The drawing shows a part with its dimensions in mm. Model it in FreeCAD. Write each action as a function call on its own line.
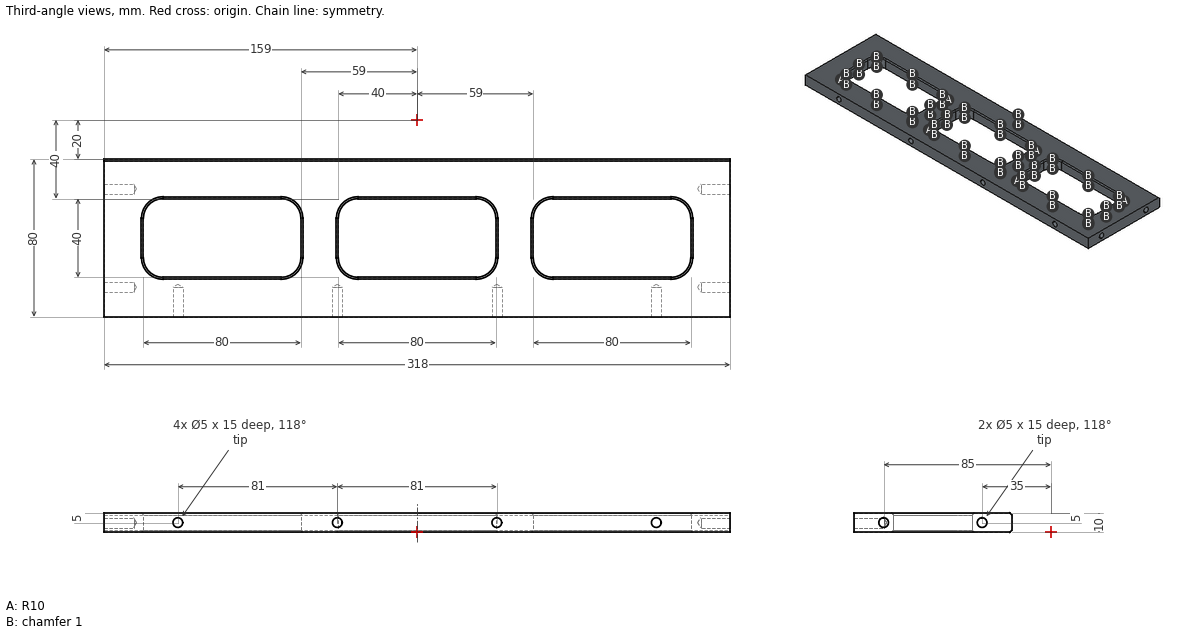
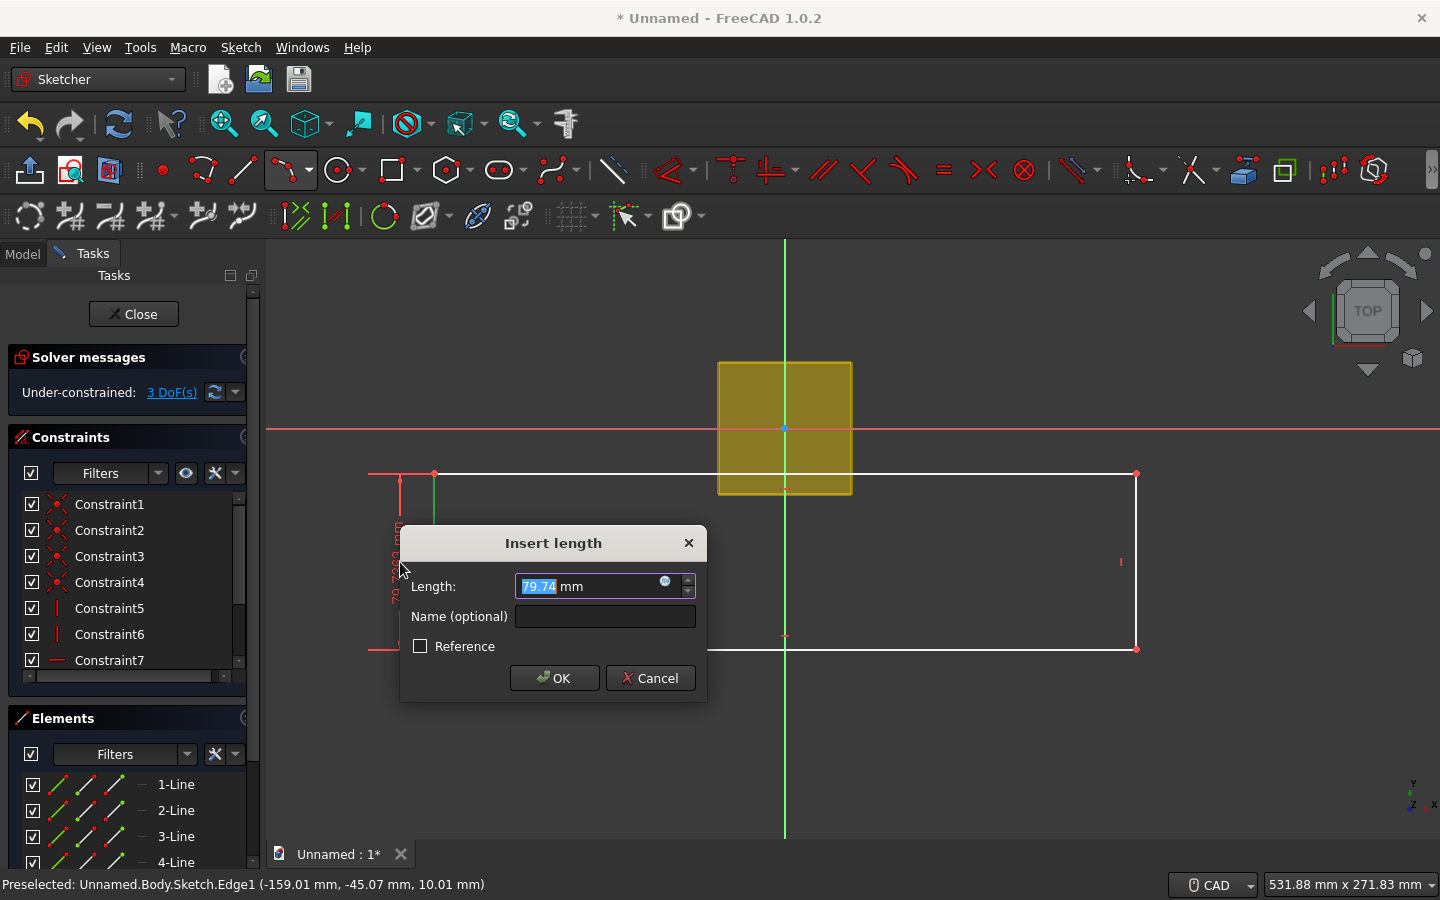
text(80)
key(Return)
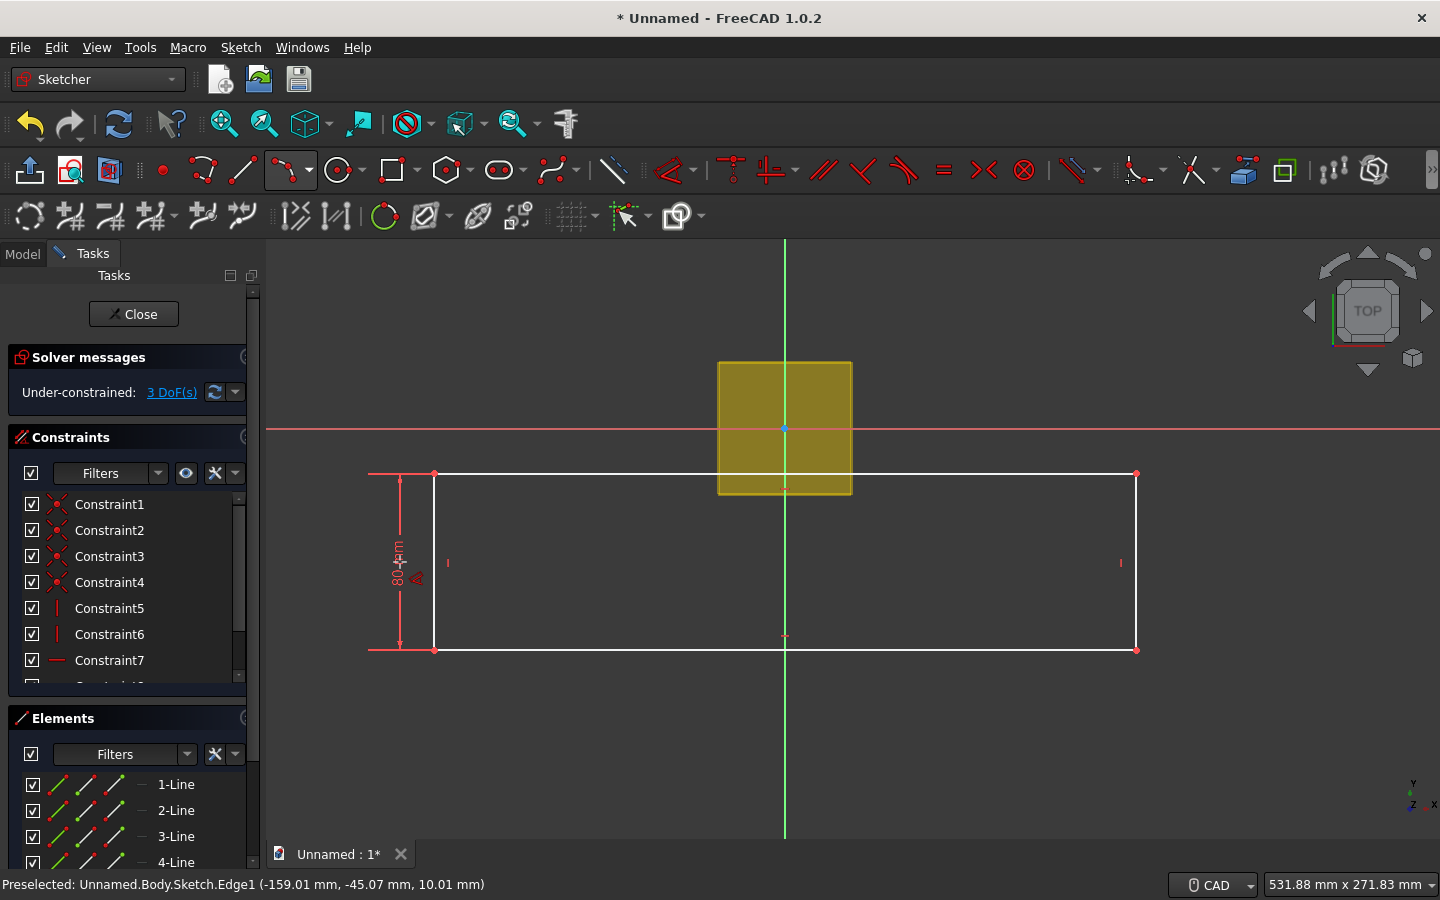
click(645, 650)
click(624, 684)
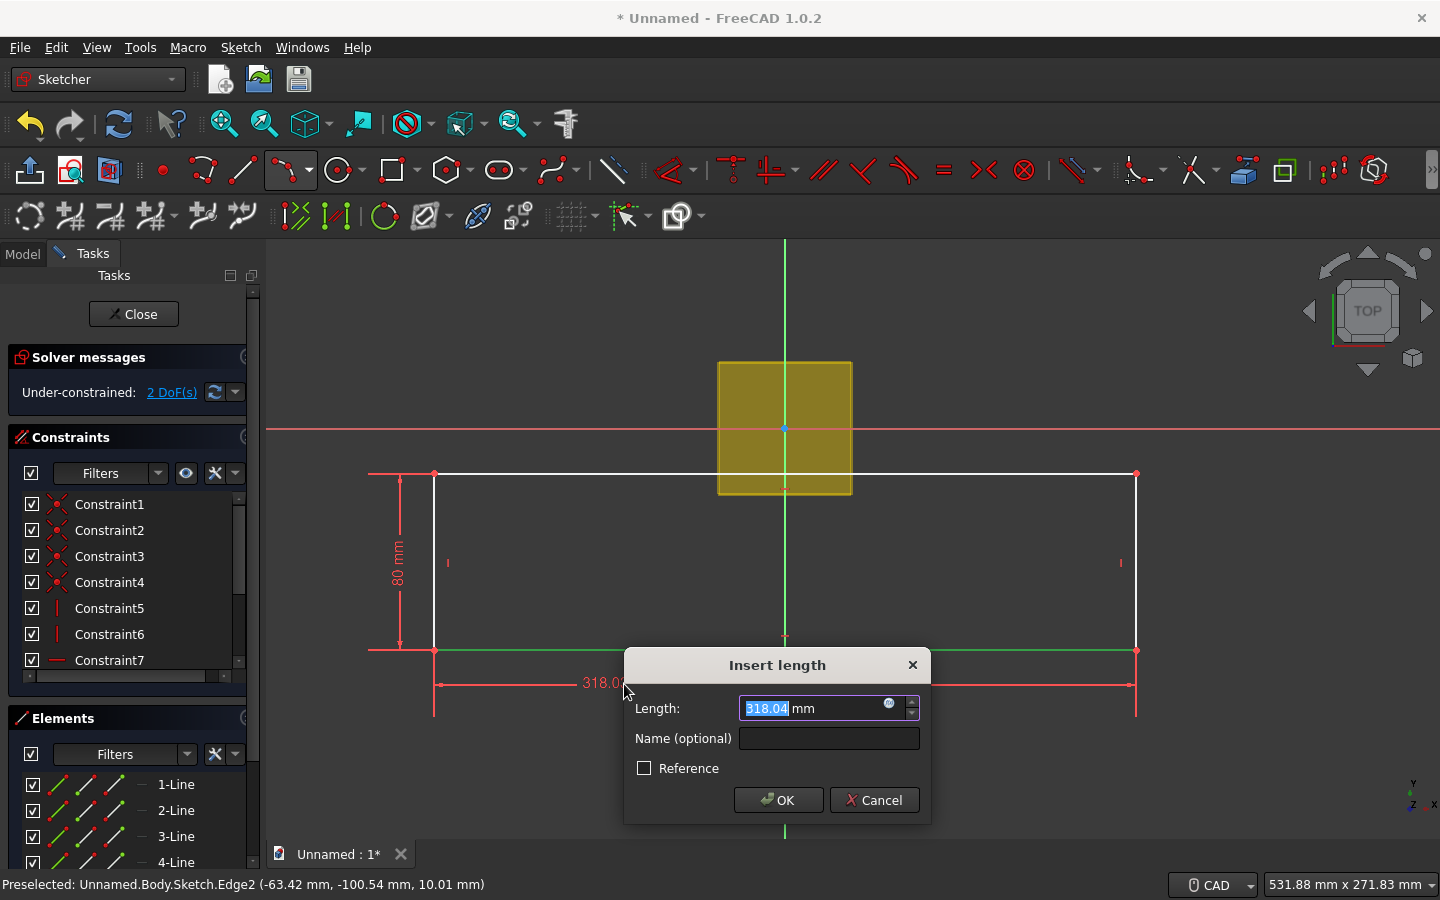
text(318)
key(Return)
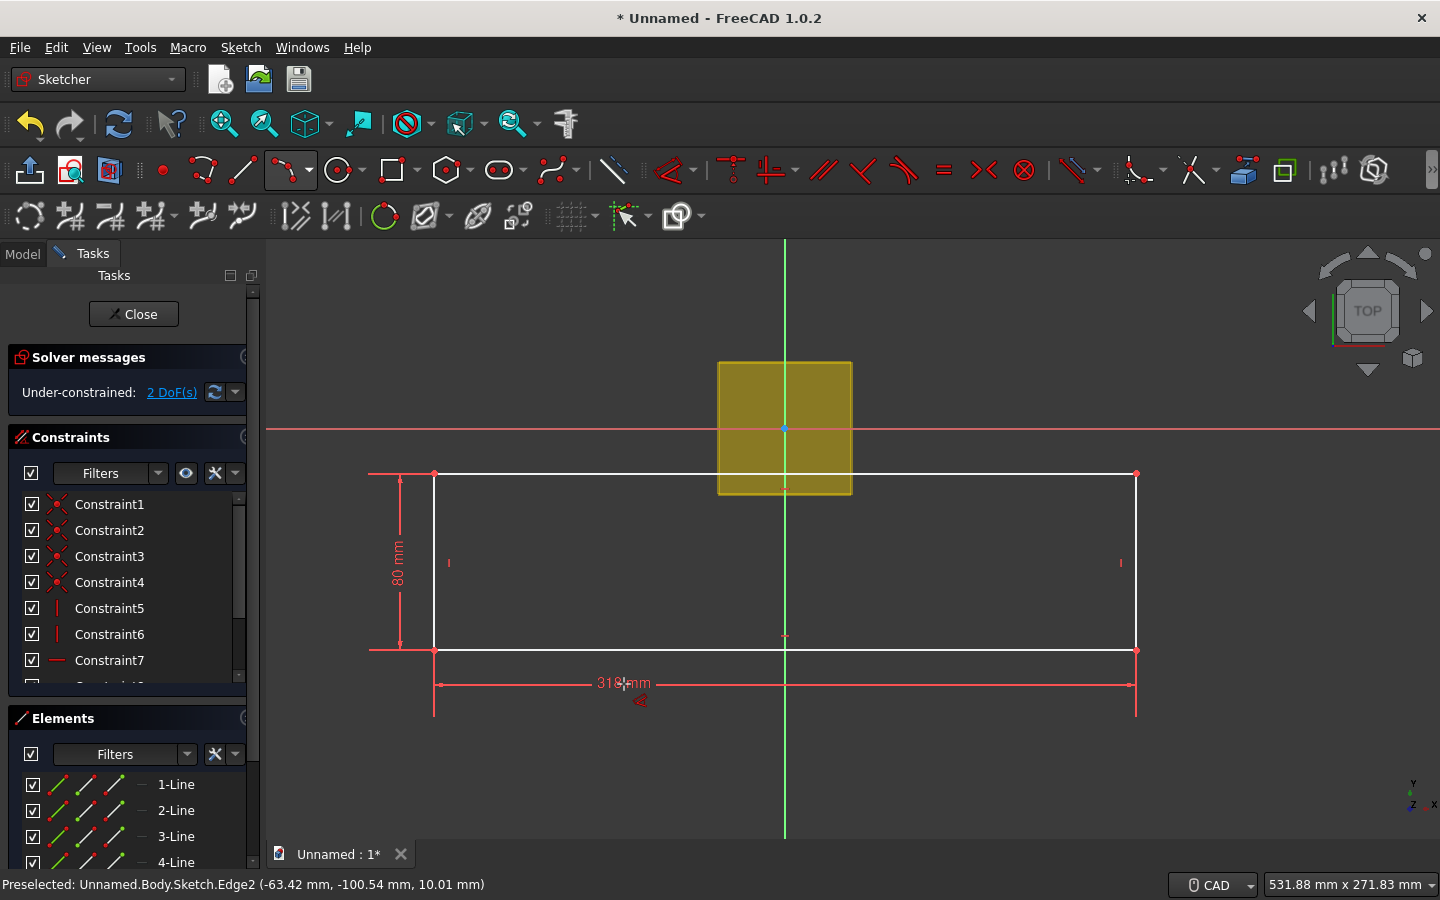
click(434, 474)
click(400, 451)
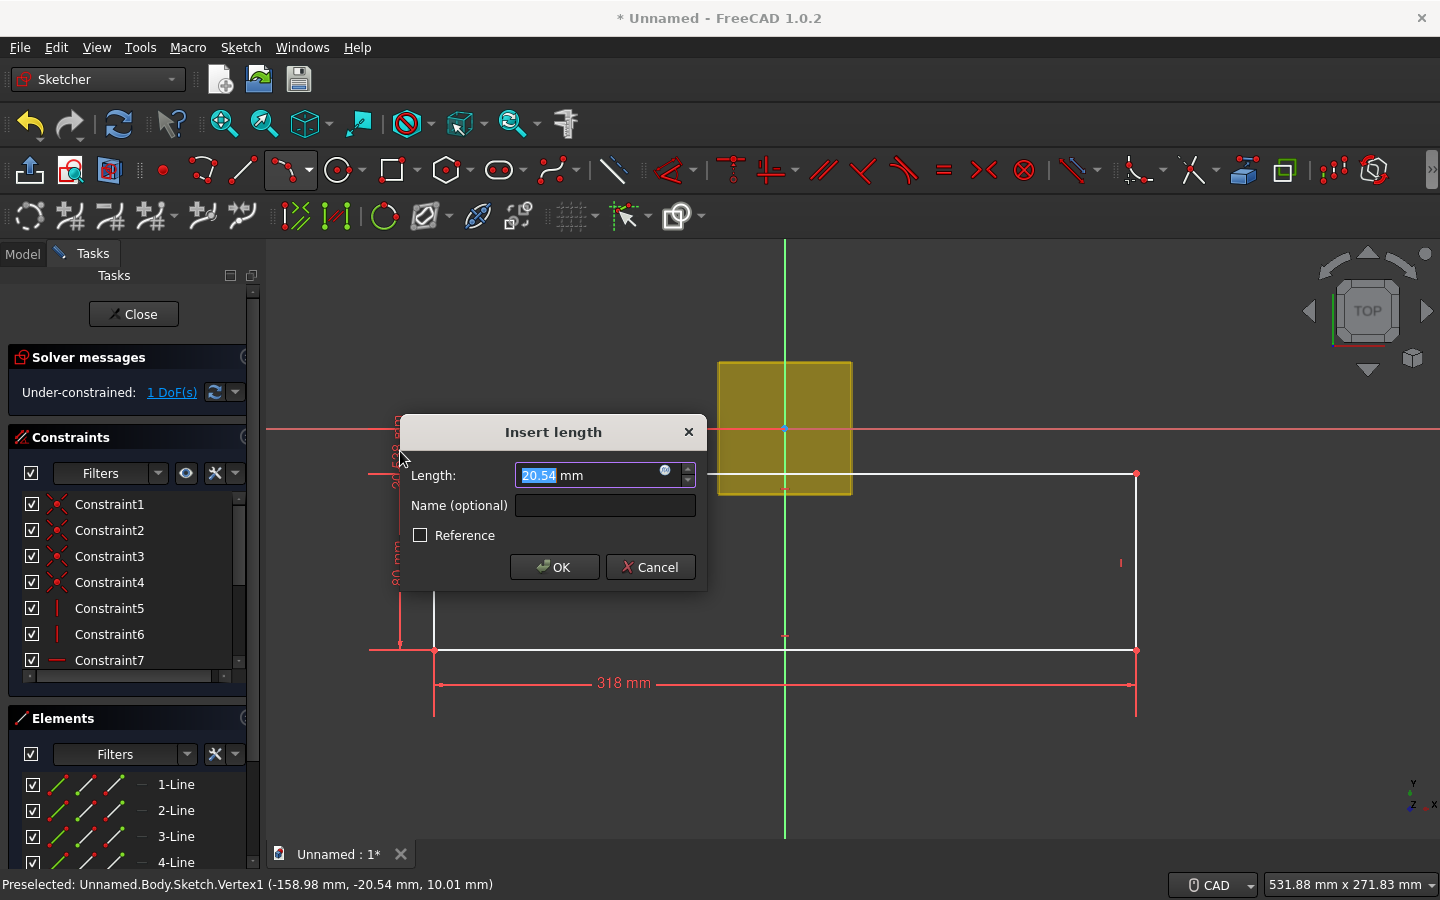
text(20)
key(Return)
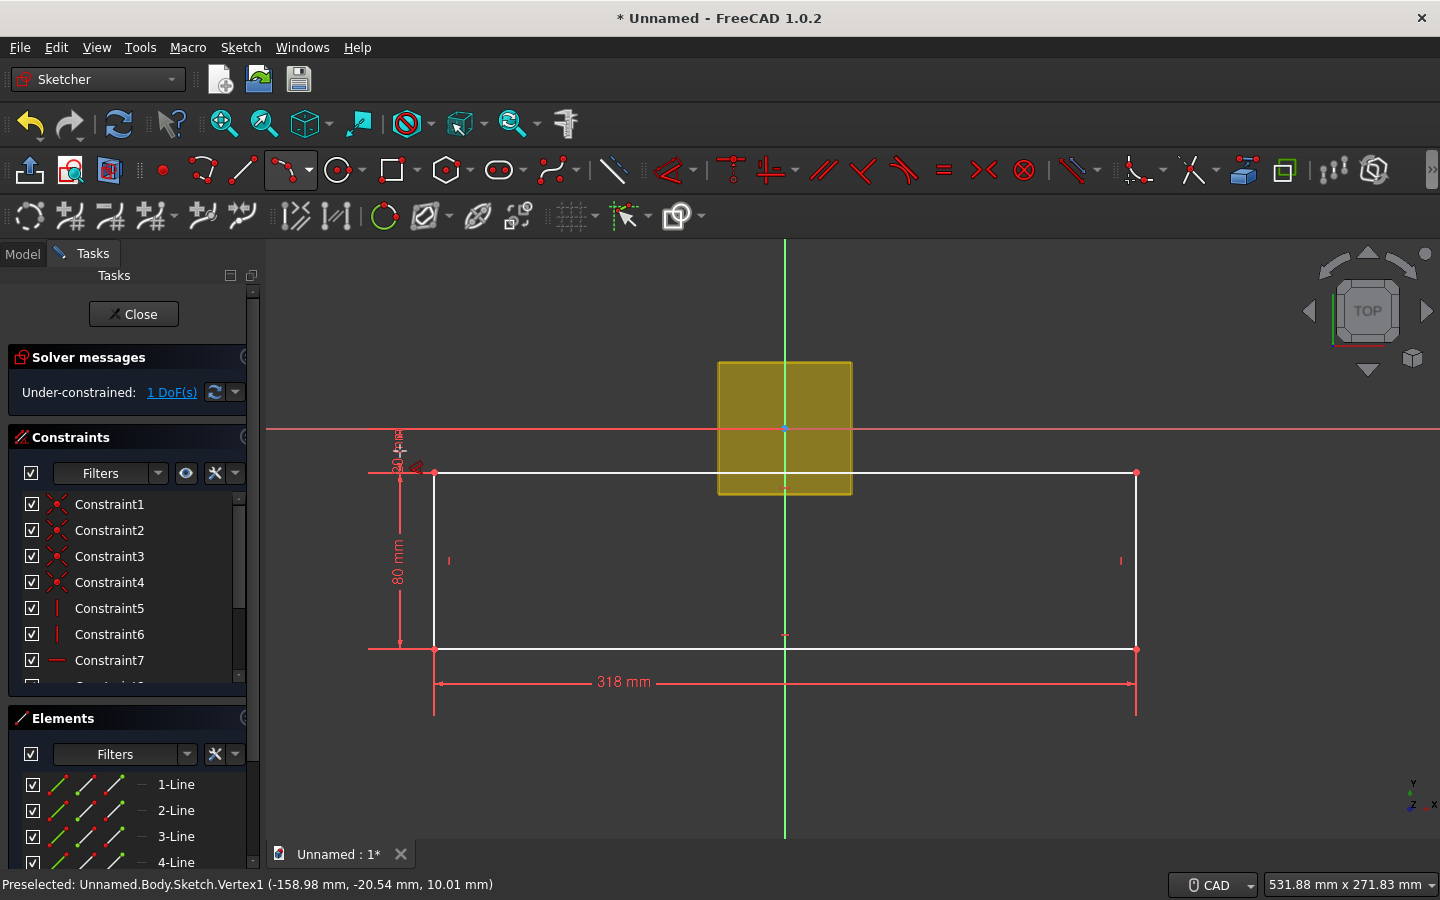
click(434, 473)
click(610, 395)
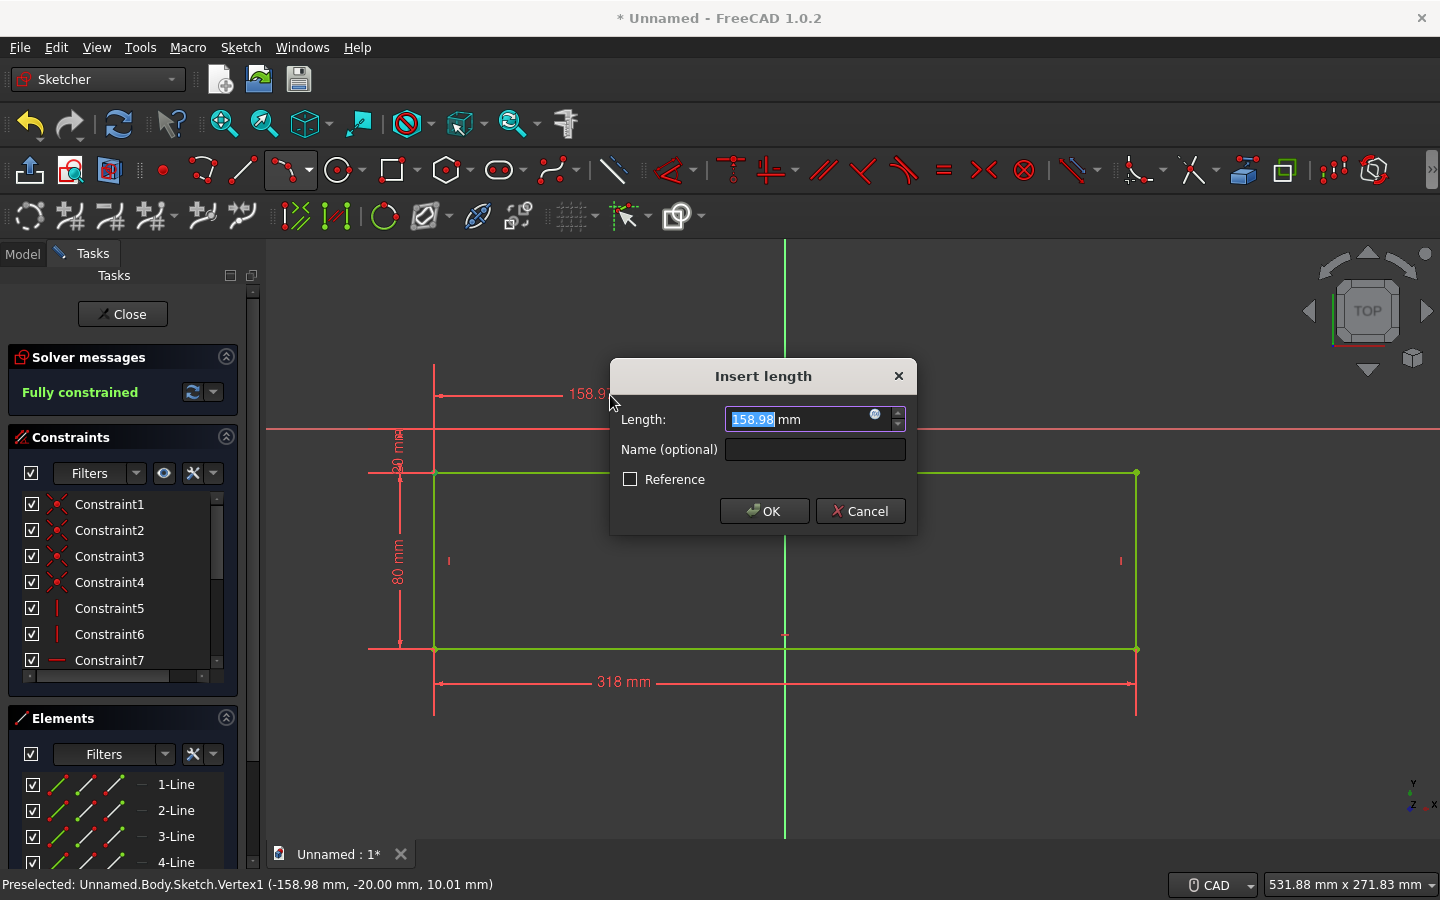
text(159)
key(Return)
key(Escape)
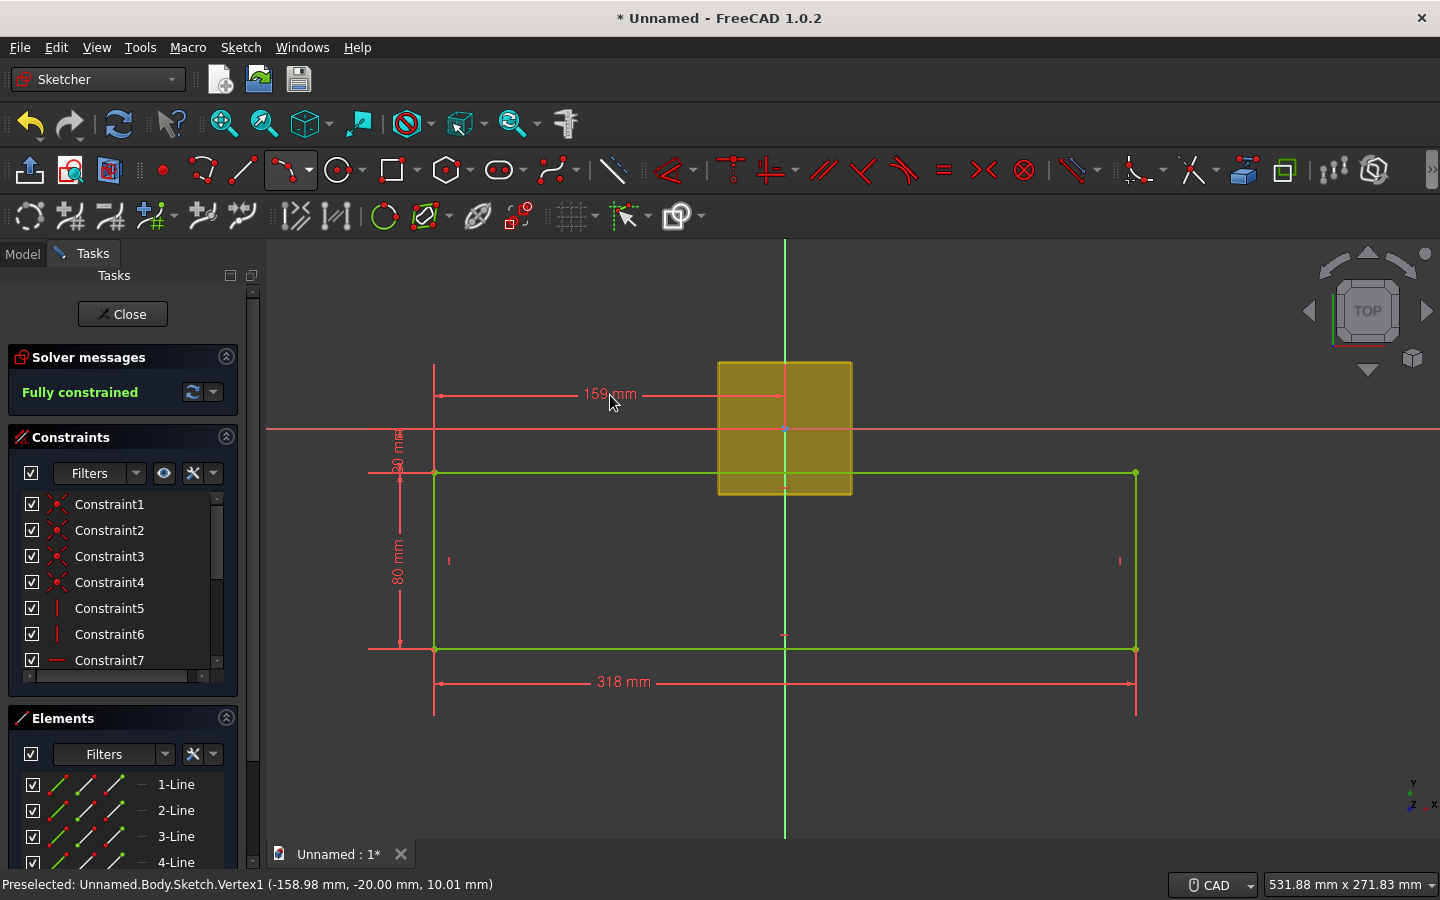
click(123, 314)